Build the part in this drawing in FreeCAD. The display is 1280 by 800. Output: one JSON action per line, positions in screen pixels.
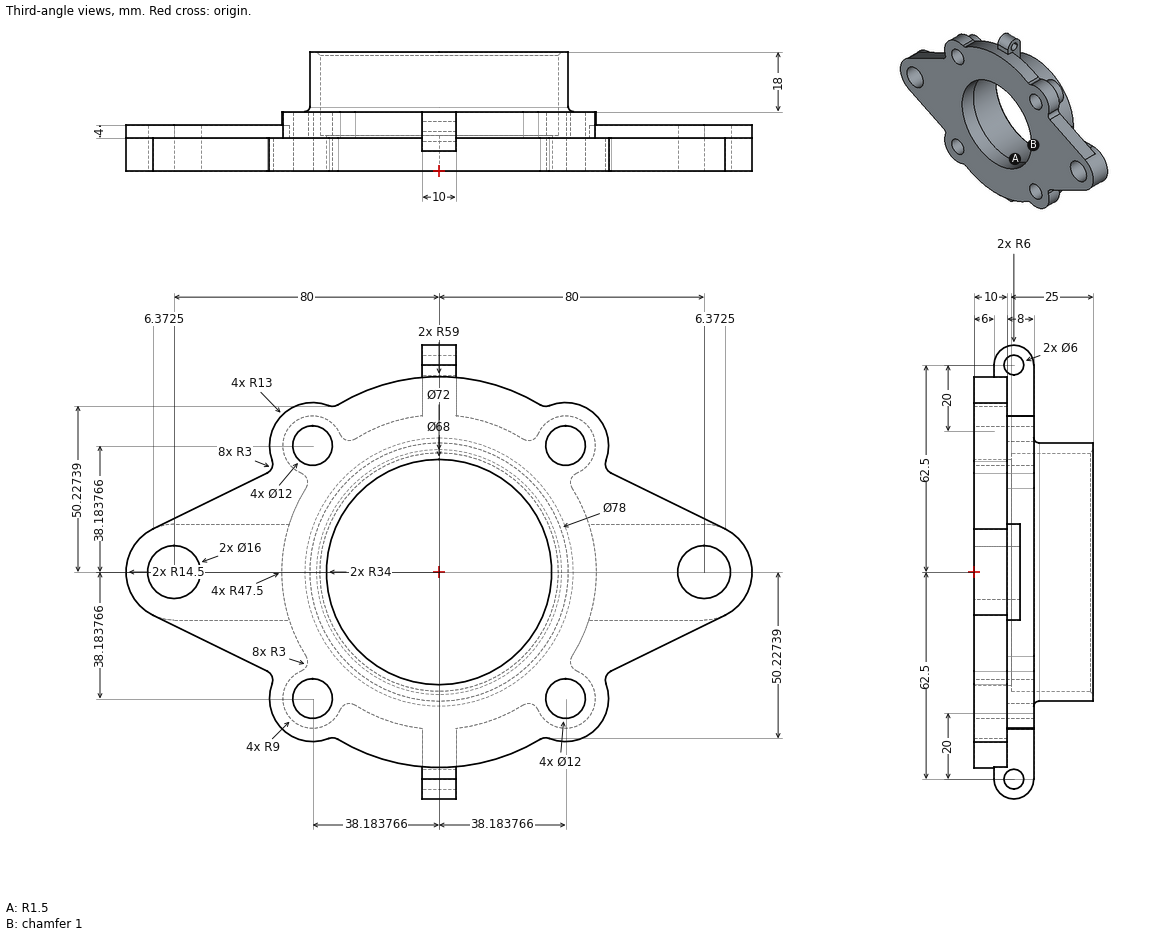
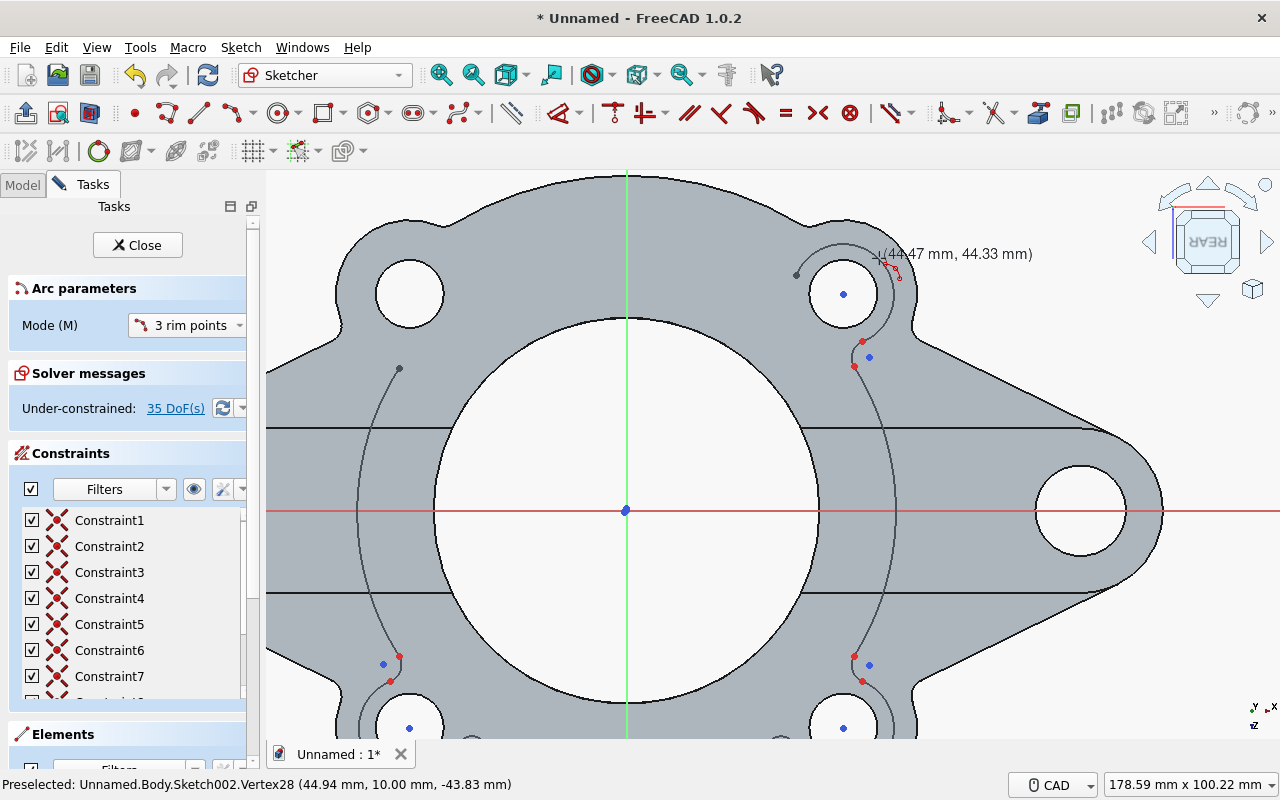
{"action": "left_click", "coordinate": [796, 276]}
{"action": "left_click", "coordinate": [771, 283]}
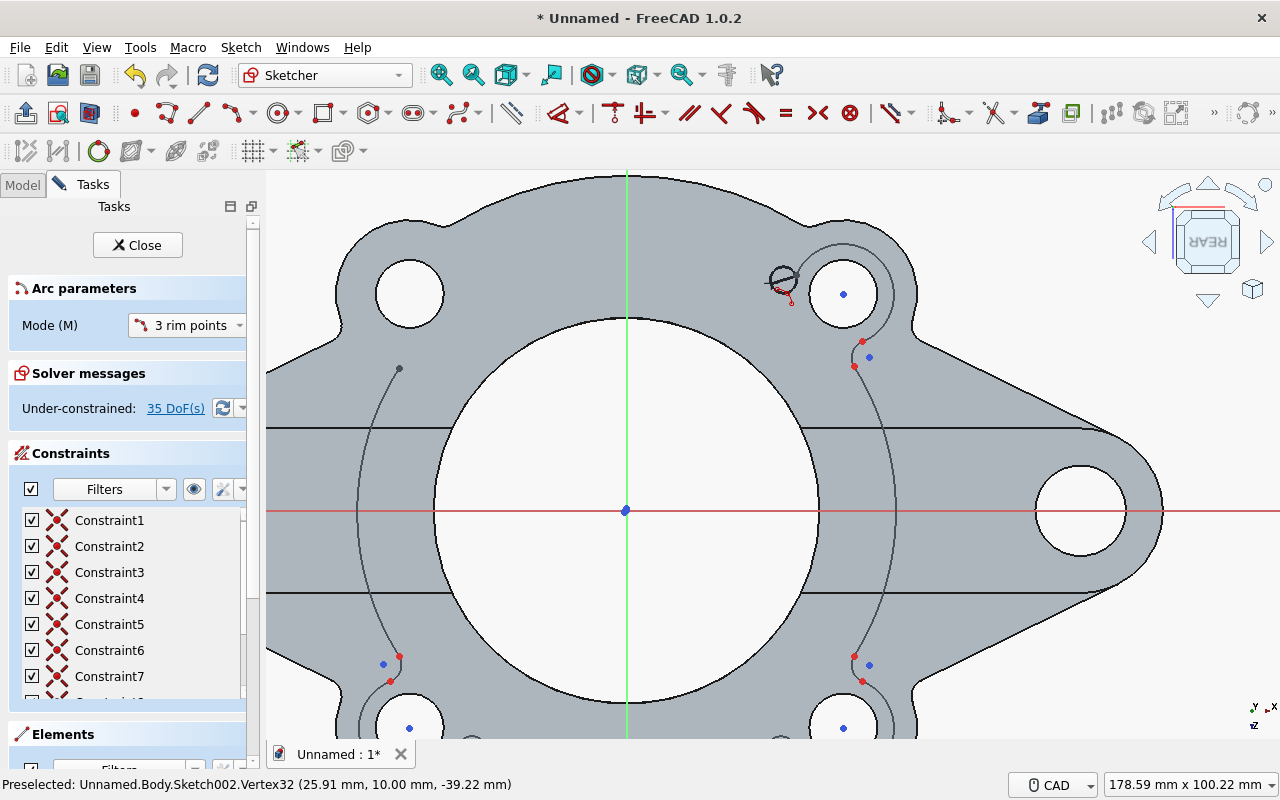
{"action": "scroll", "coordinate": [785, 285], "scroll_direction": "up", "scroll_amount": 5}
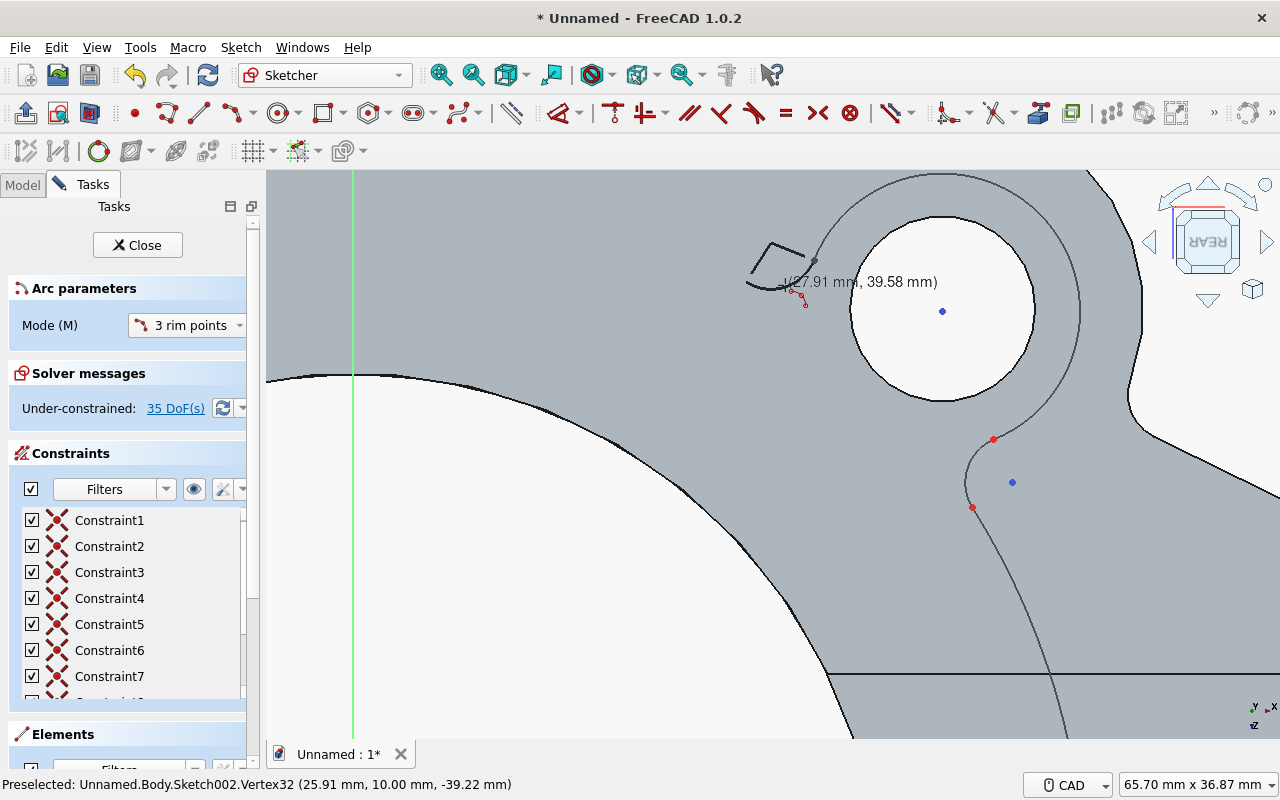
{"action": "left_click", "coordinate": [785, 284]}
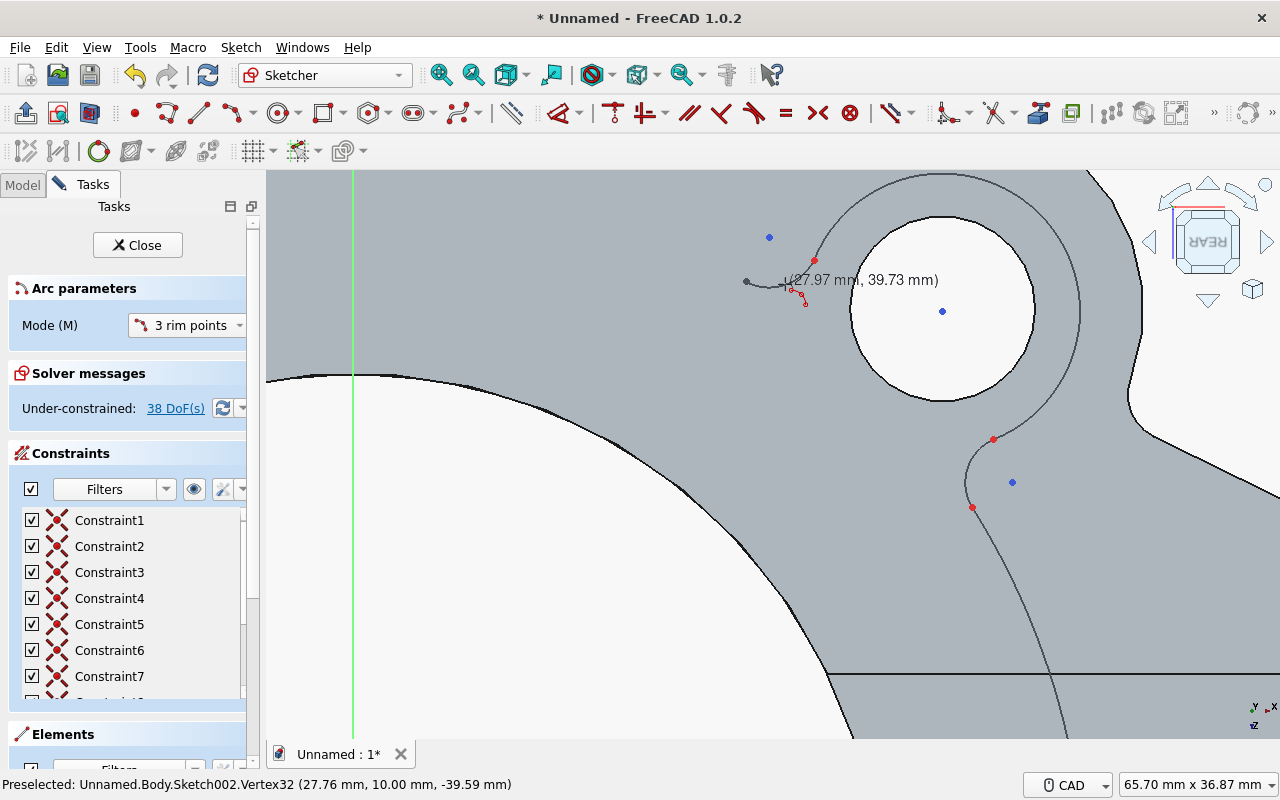
{"action": "scroll", "coordinate": [819, 309], "scroll_direction": "down", "scroll_amount": 7}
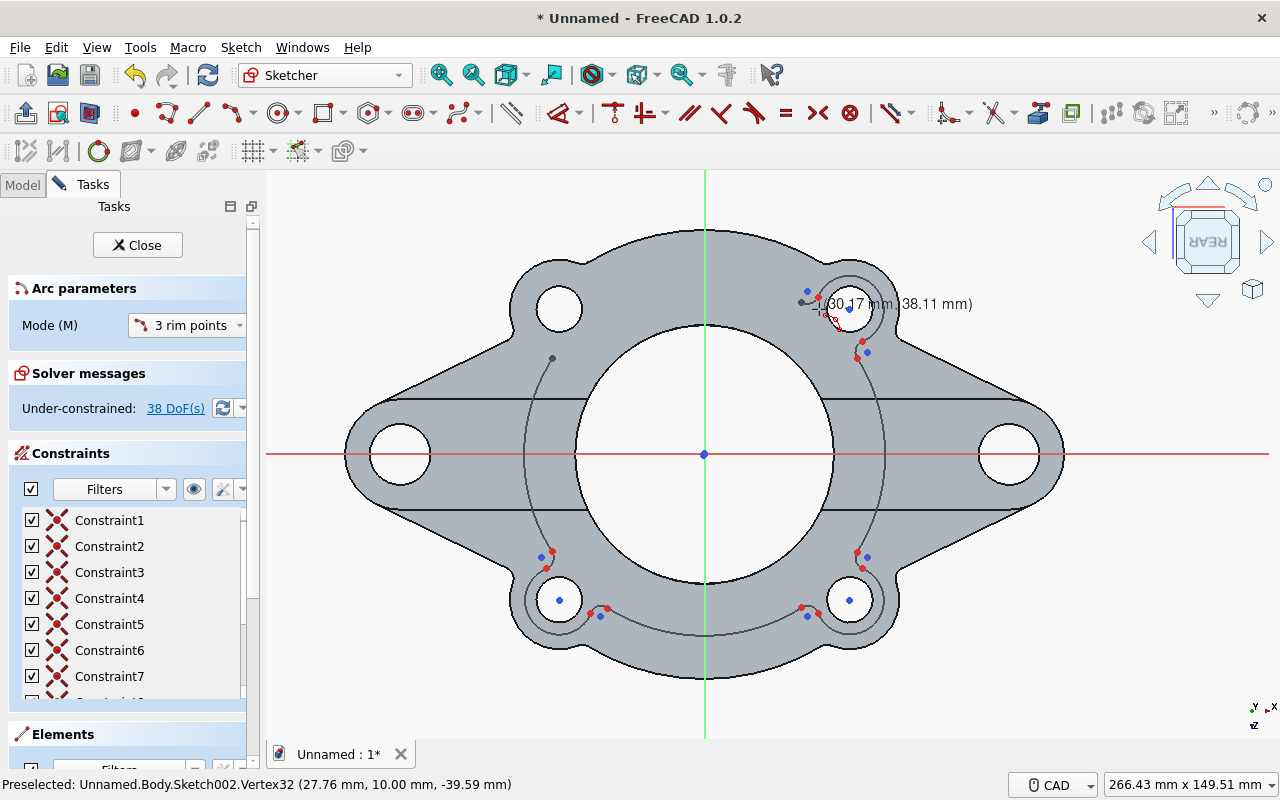
{"action": "scroll", "coordinate": [801, 302], "scroll_direction": "up", "scroll_amount": 2}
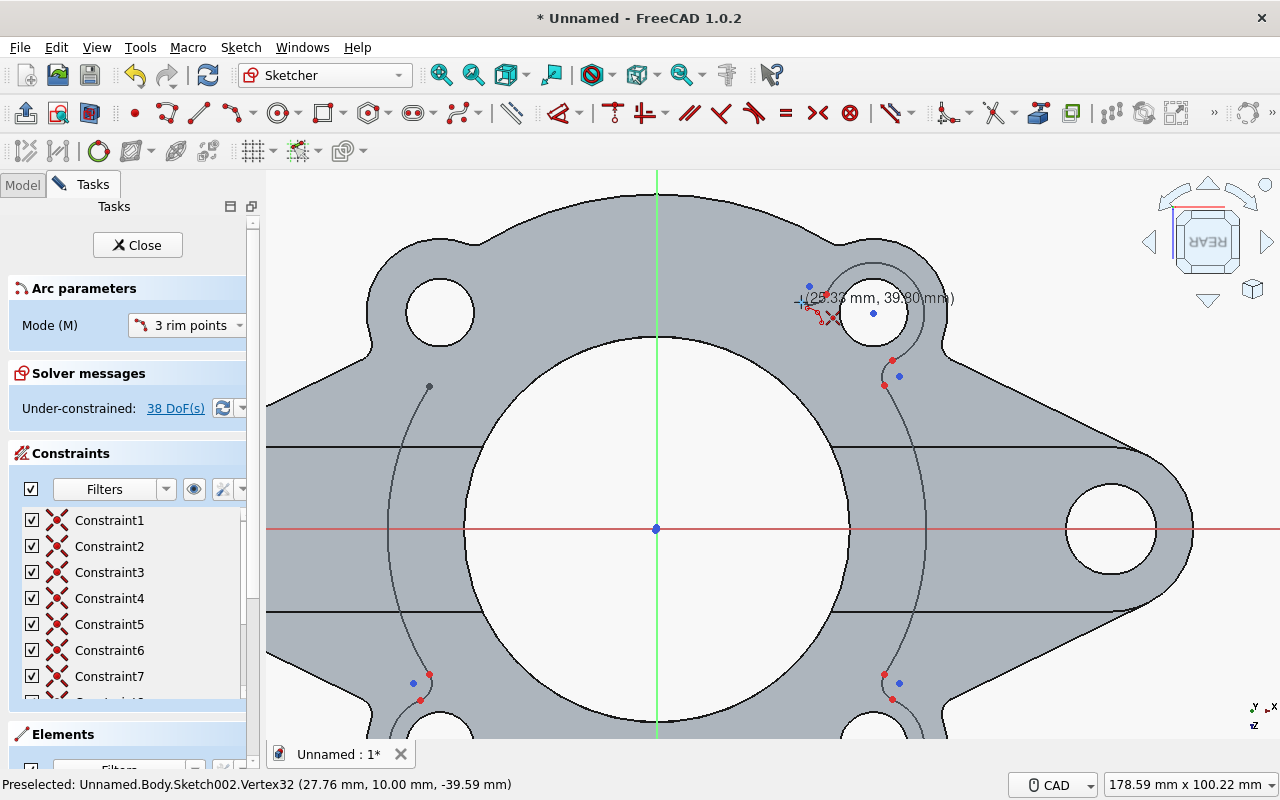
{"action": "left_click", "coordinate": [801, 303]}
{"action": "left_click", "coordinate": [512, 302]}
{"action": "left_click", "coordinate": [687, 261]}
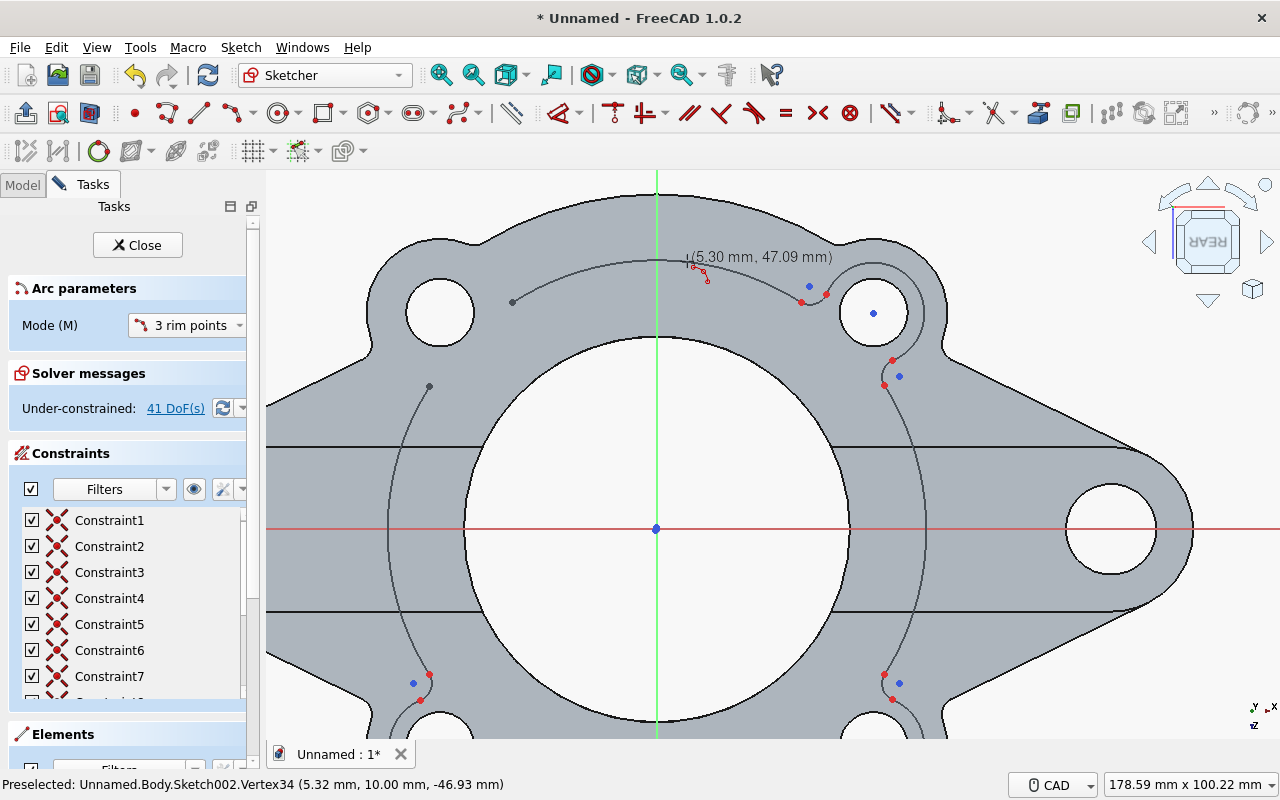
{"action": "left_click", "coordinate": [512, 303]}
{"action": "left_click", "coordinate": [488, 294]}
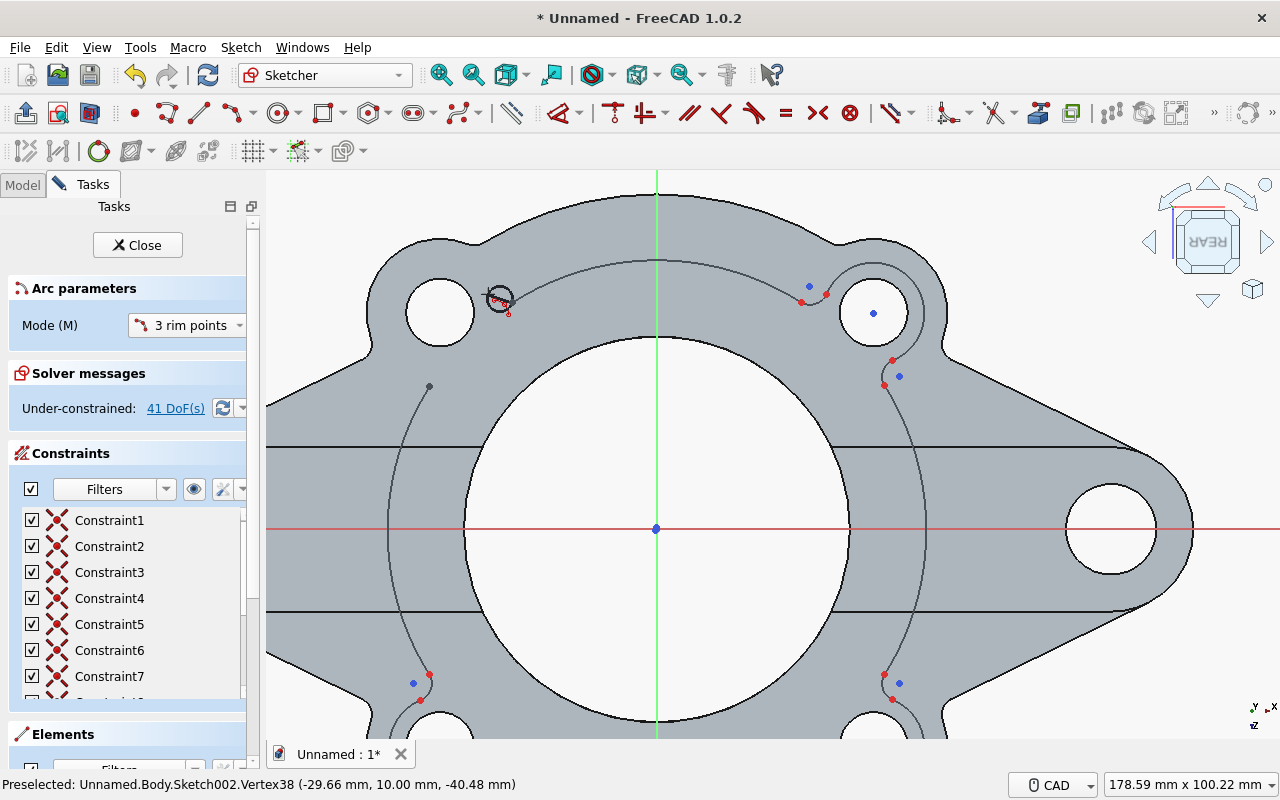
{"action": "scroll", "coordinate": [498, 303], "scroll_direction": "up", "scroll_amount": 5}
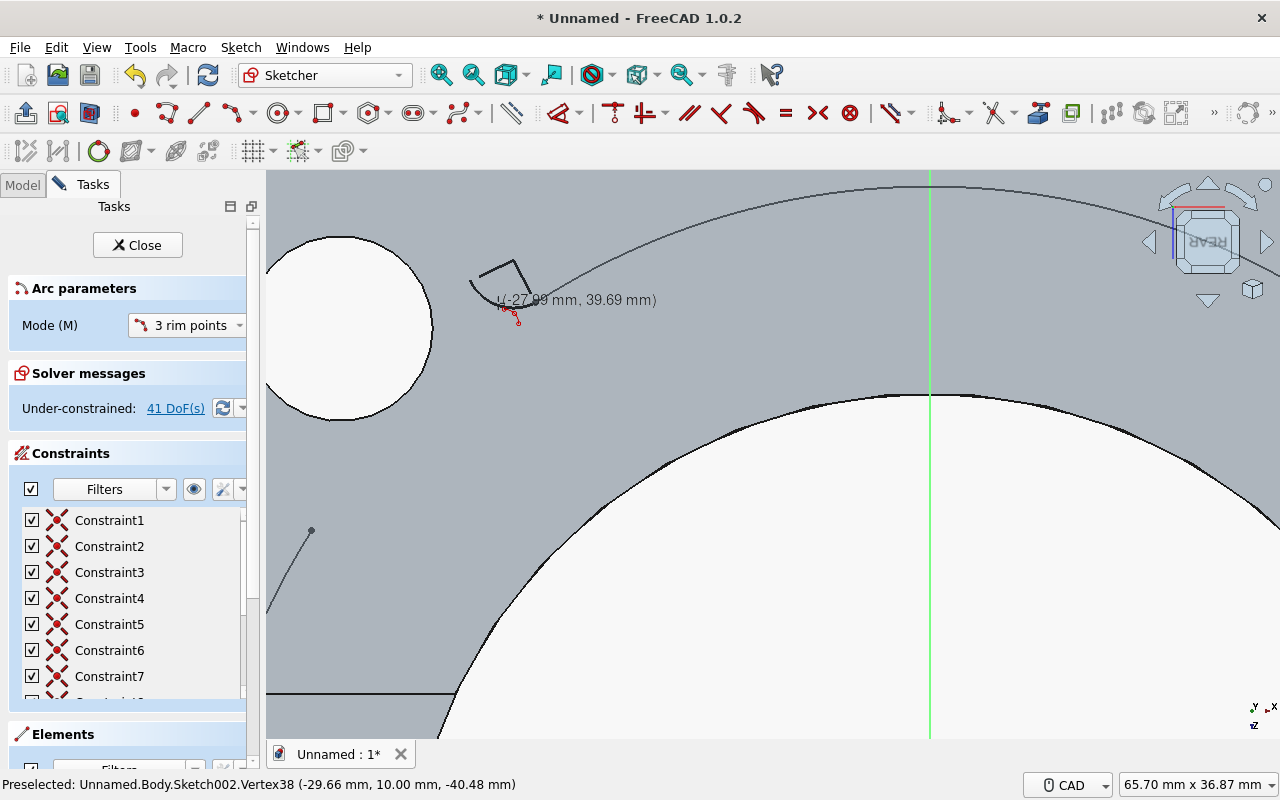
{"action": "left_click", "coordinate": [498, 304]}